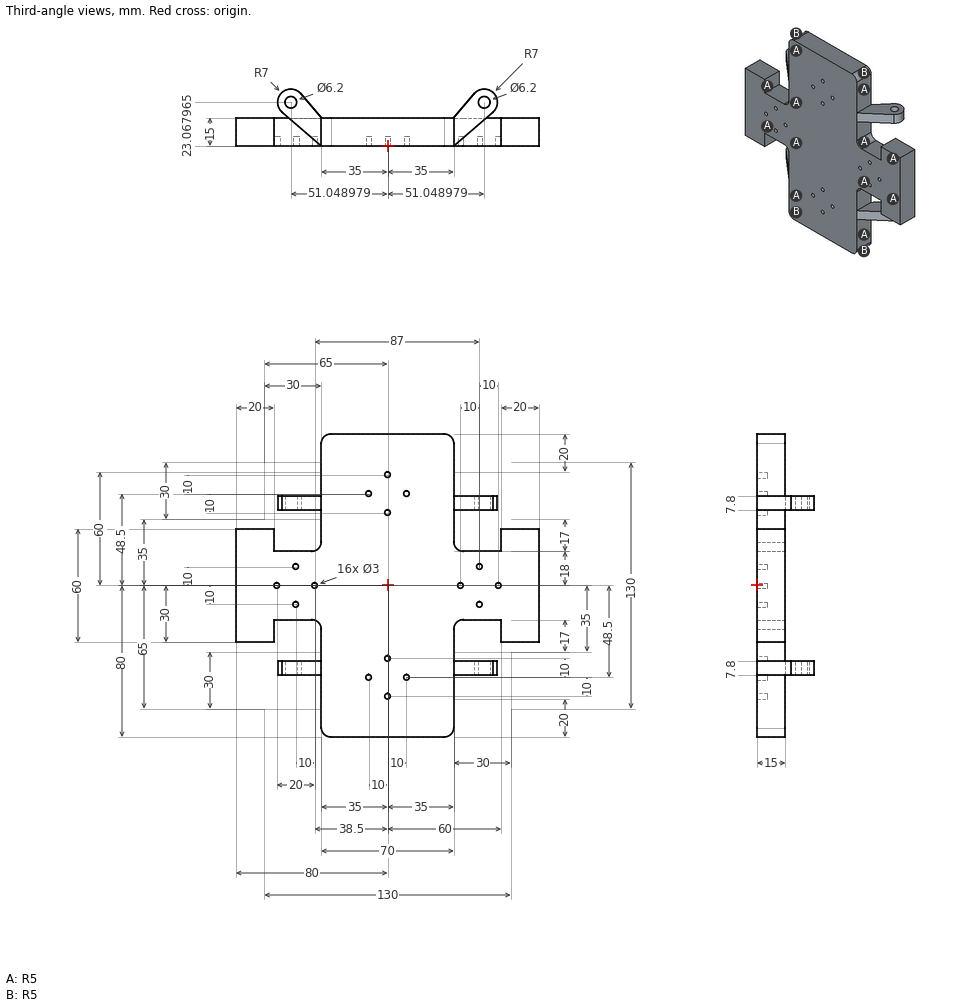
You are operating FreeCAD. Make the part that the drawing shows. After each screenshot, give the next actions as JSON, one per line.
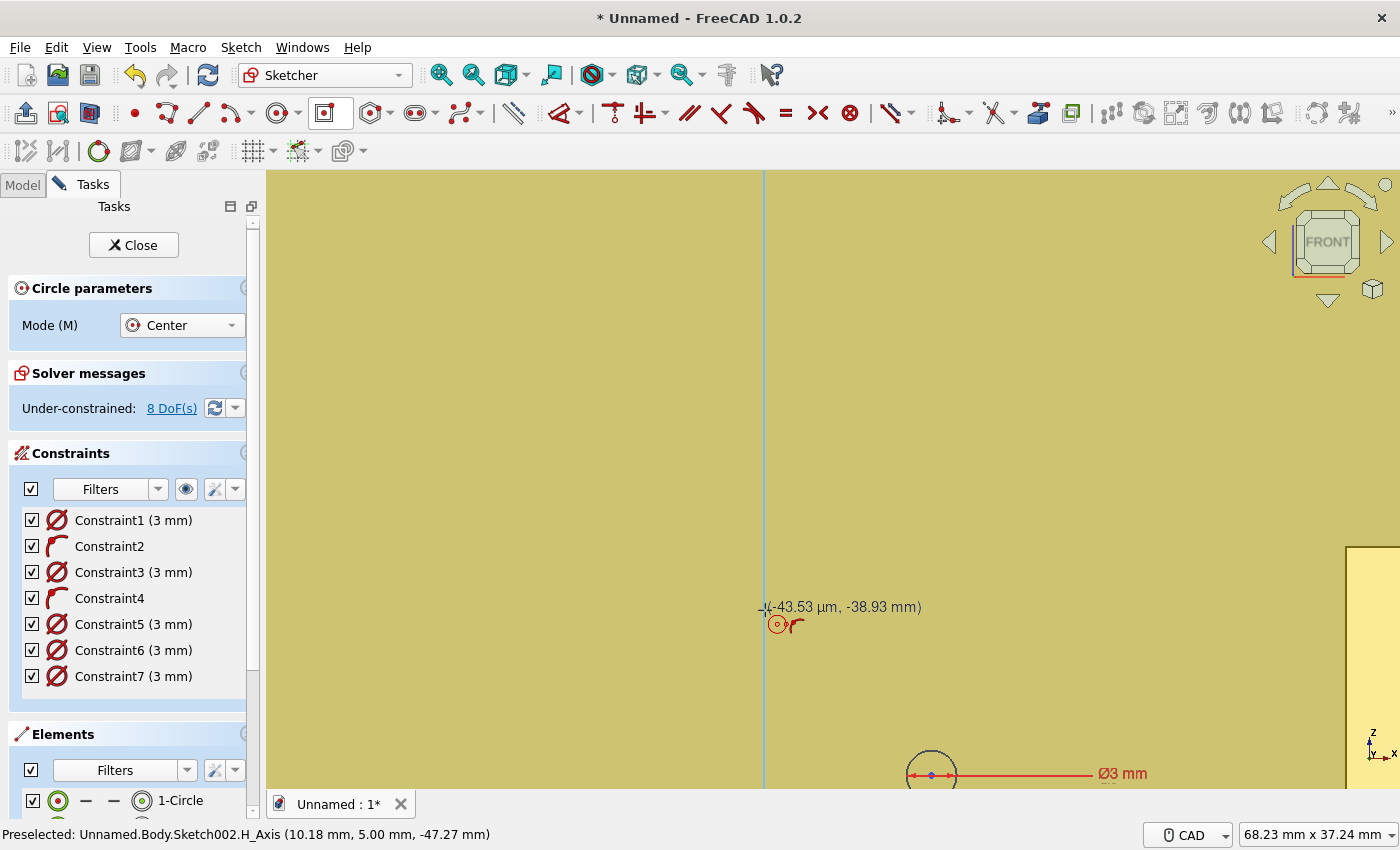
{"action": "scroll", "coordinate": [765, 610], "scroll_direction": "down", "scroll_amount": 8}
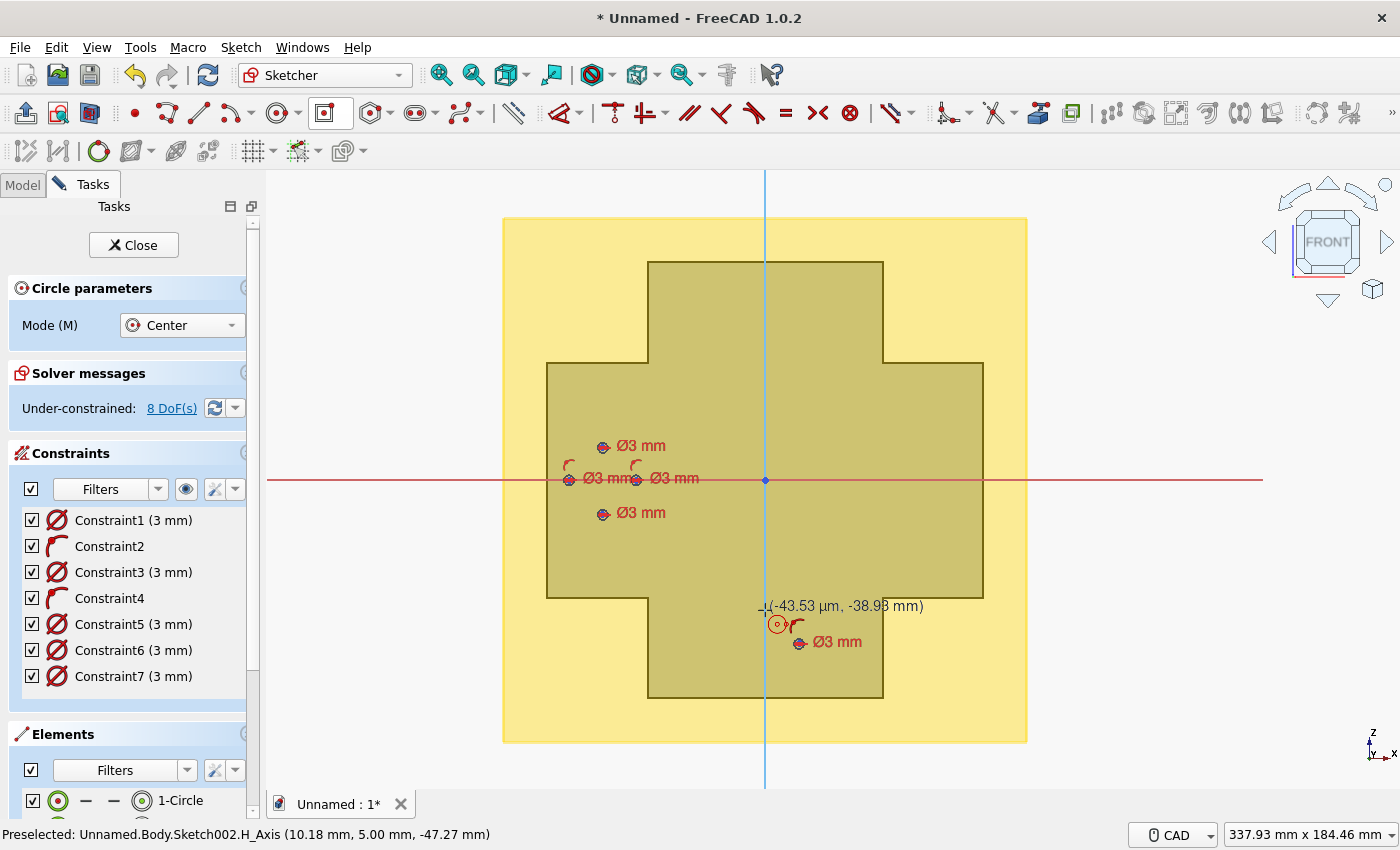
{"action": "left_click", "coordinate": [765, 610]}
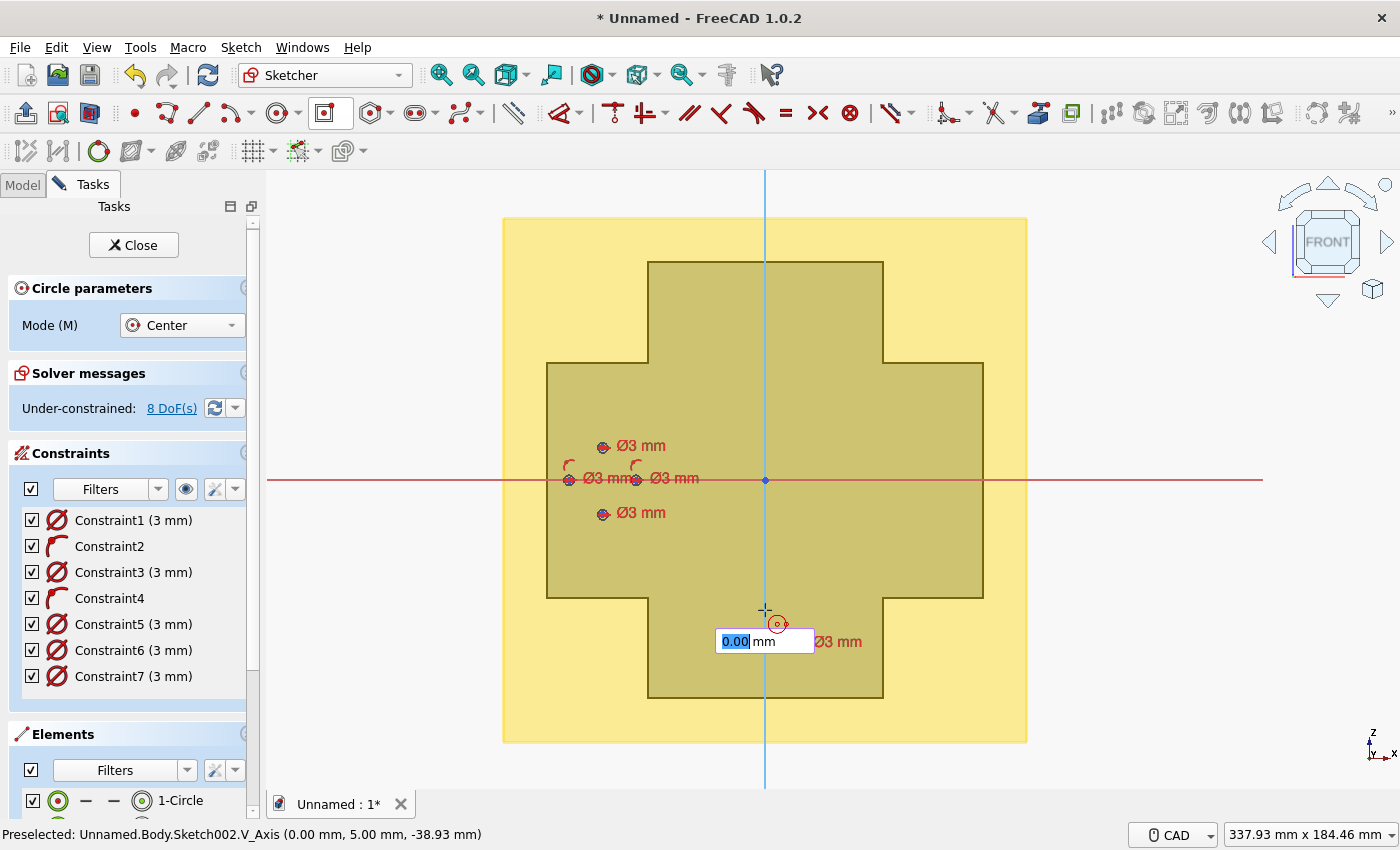
{"action": "scroll", "coordinate": [770, 608], "scroll_direction": "up", "scroll_amount": 7}
{"action": "mouse_move", "coordinate": [768, 605]}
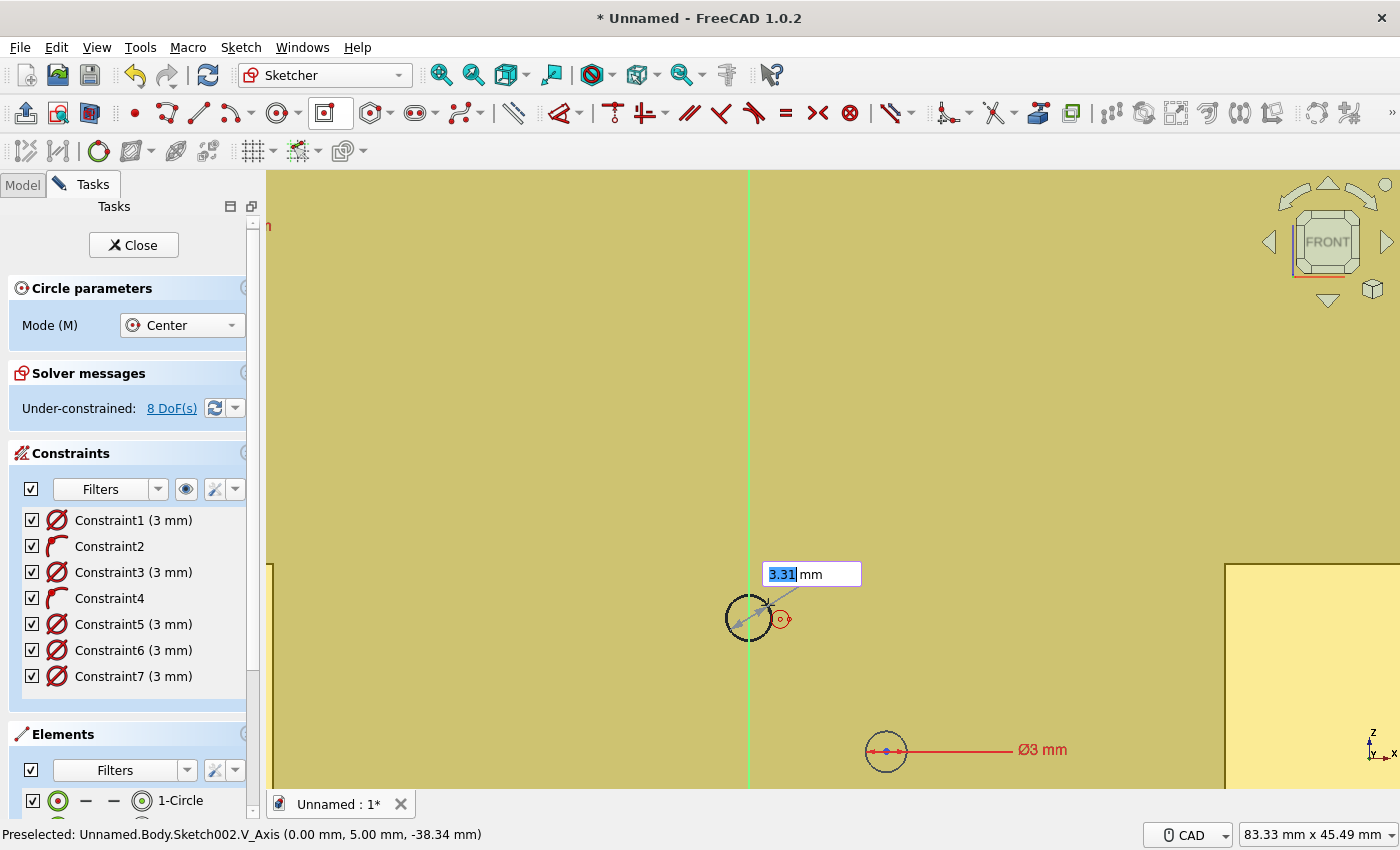
{"action": "type", "text": "3"}
{"action": "key", "text": "Return"}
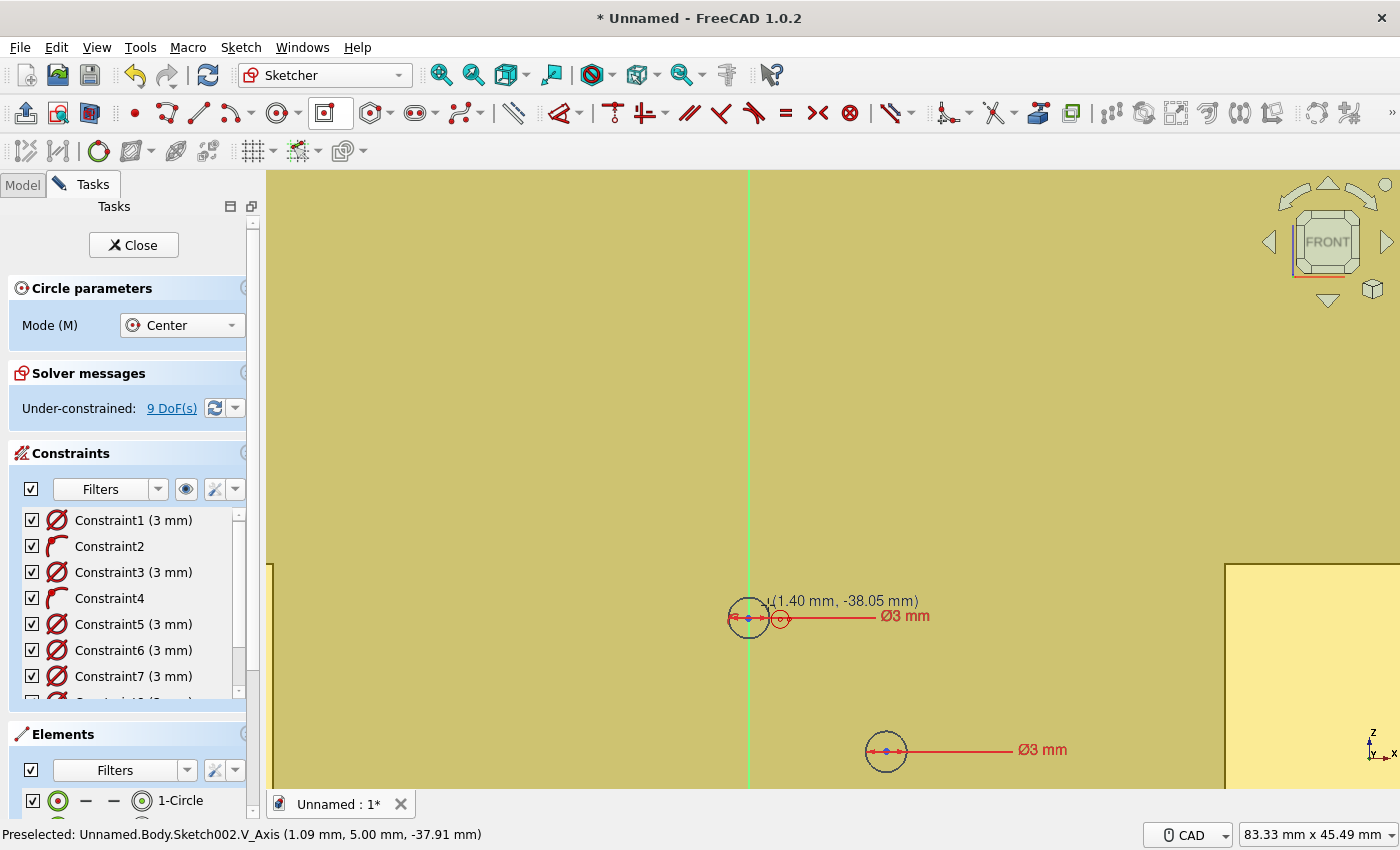
{"action": "scroll", "coordinate": [770, 608], "scroll_direction": "down", "scroll_amount": 7}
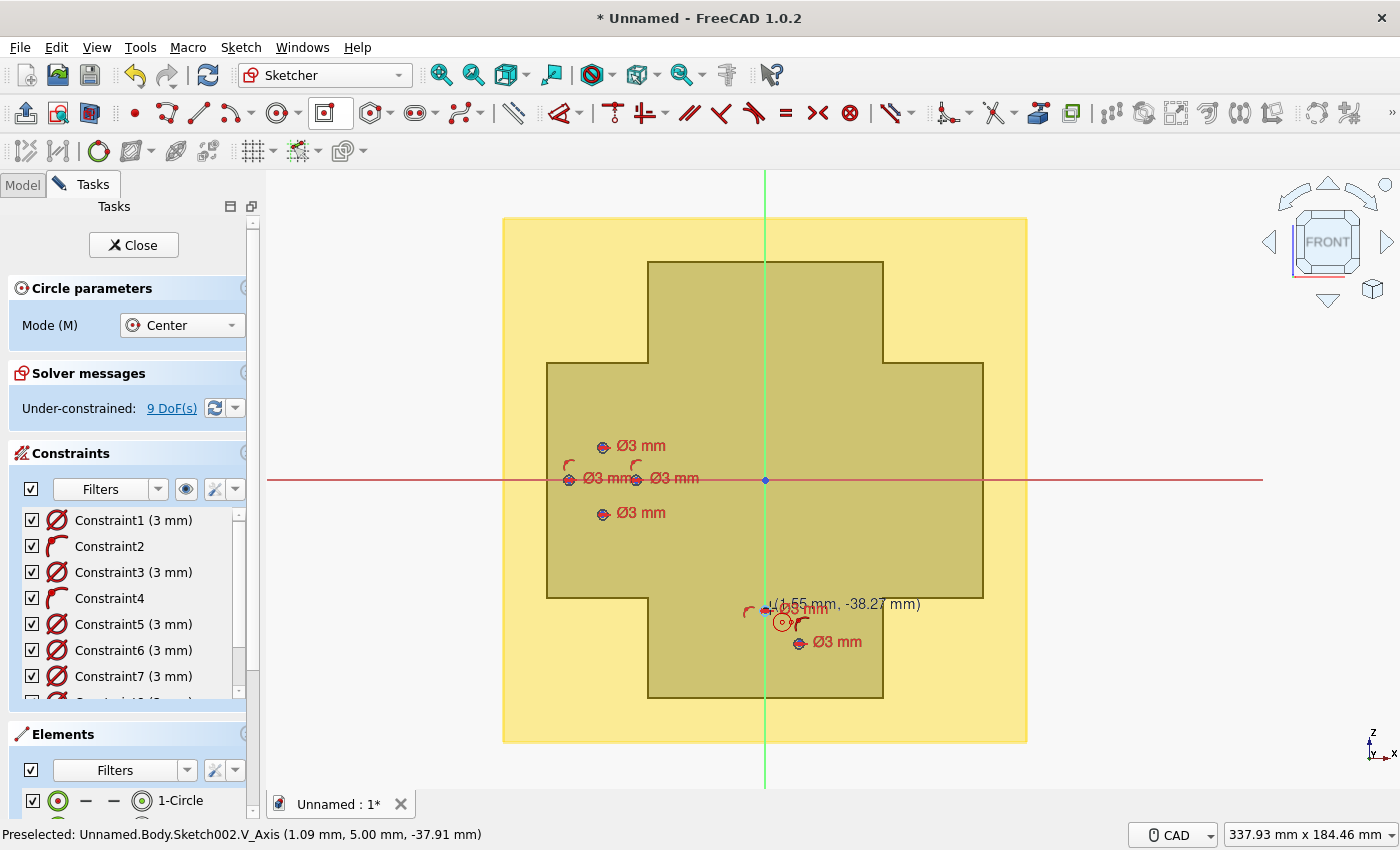
{"action": "left_click", "coordinate": [732, 643]}
{"action": "mouse_move", "coordinate": [735, 640]}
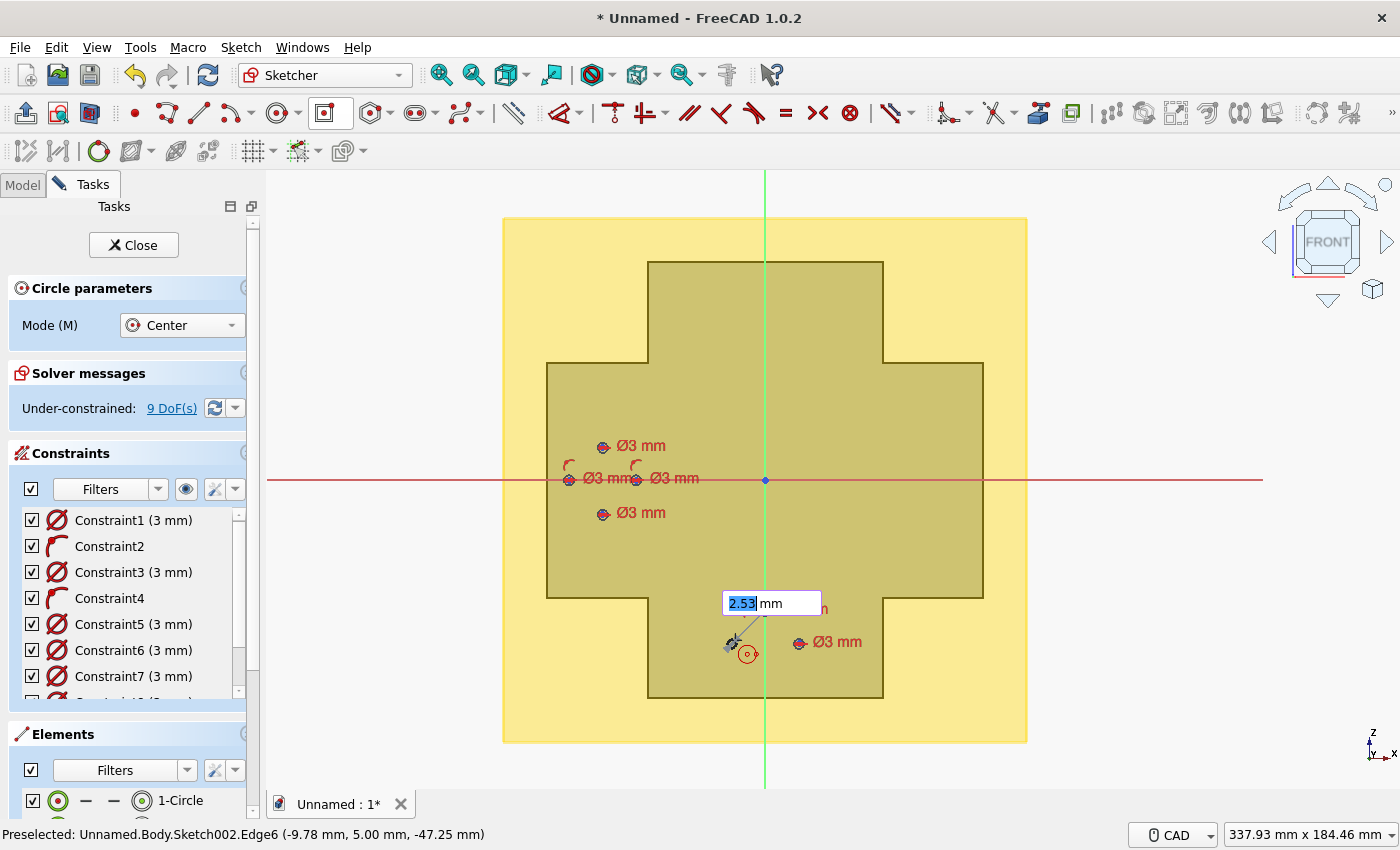
{"action": "type", "text": "3"}
{"action": "key", "text": "Return"}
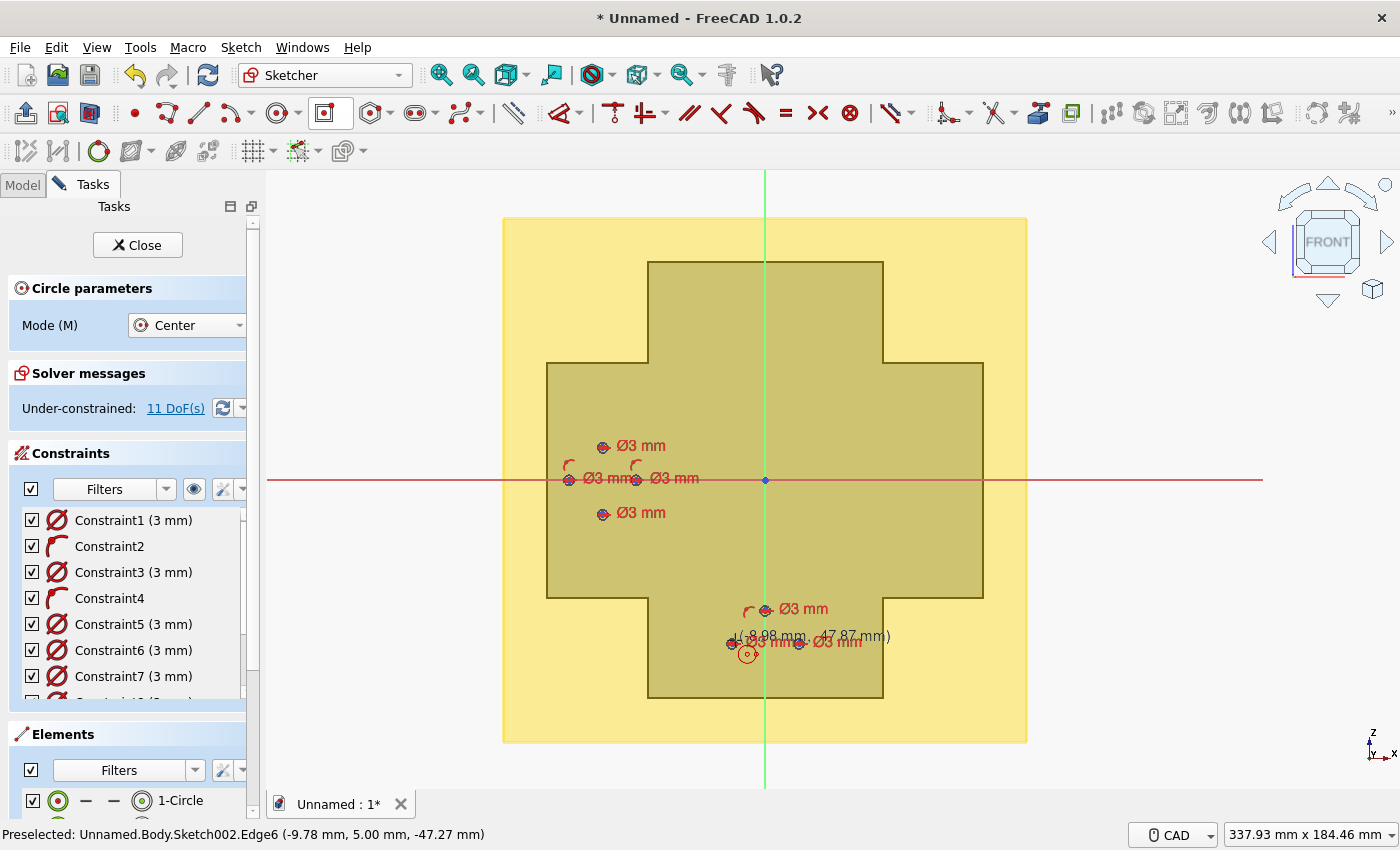
{"action": "scroll", "coordinate": [765, 677], "scroll_direction": "up", "scroll_amount": 8}